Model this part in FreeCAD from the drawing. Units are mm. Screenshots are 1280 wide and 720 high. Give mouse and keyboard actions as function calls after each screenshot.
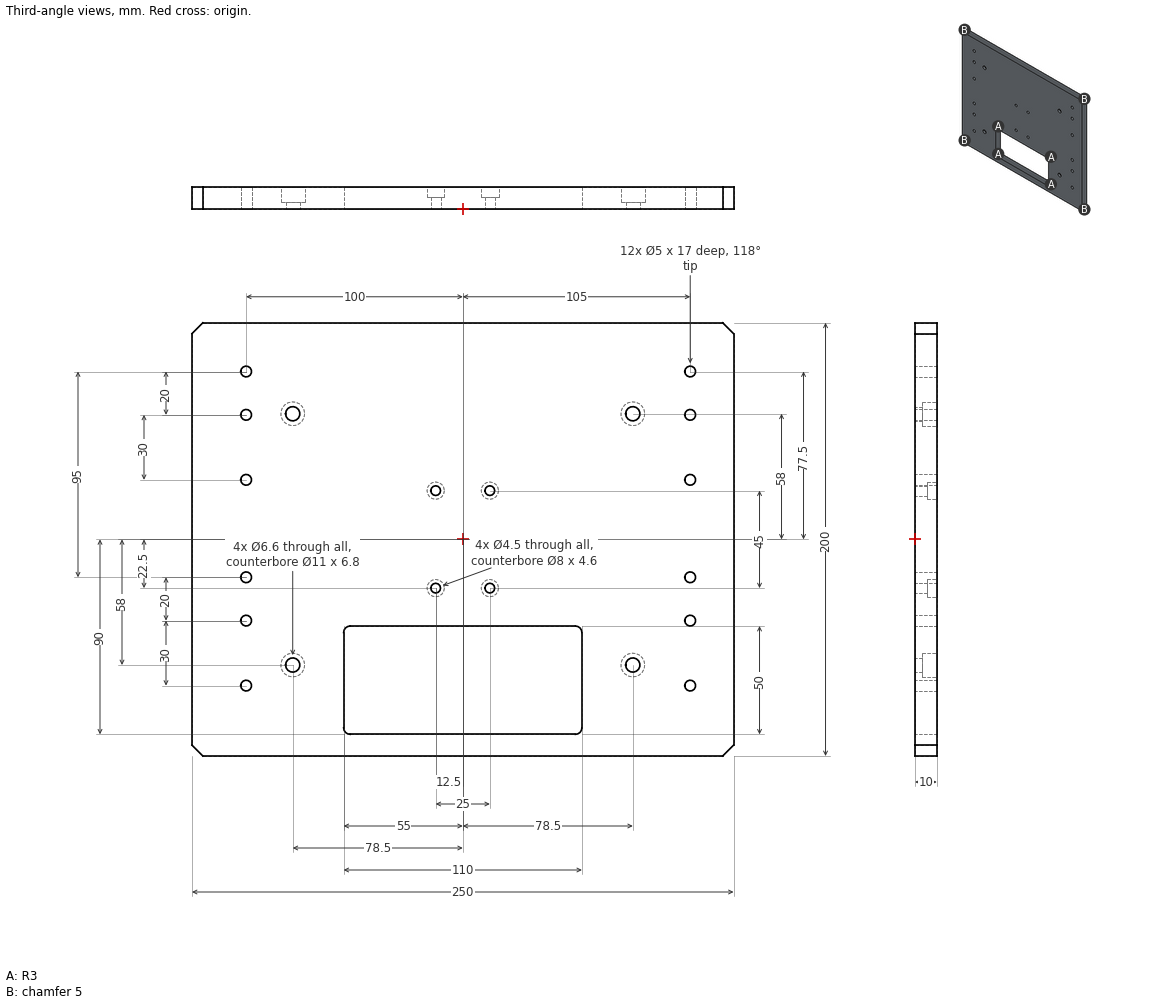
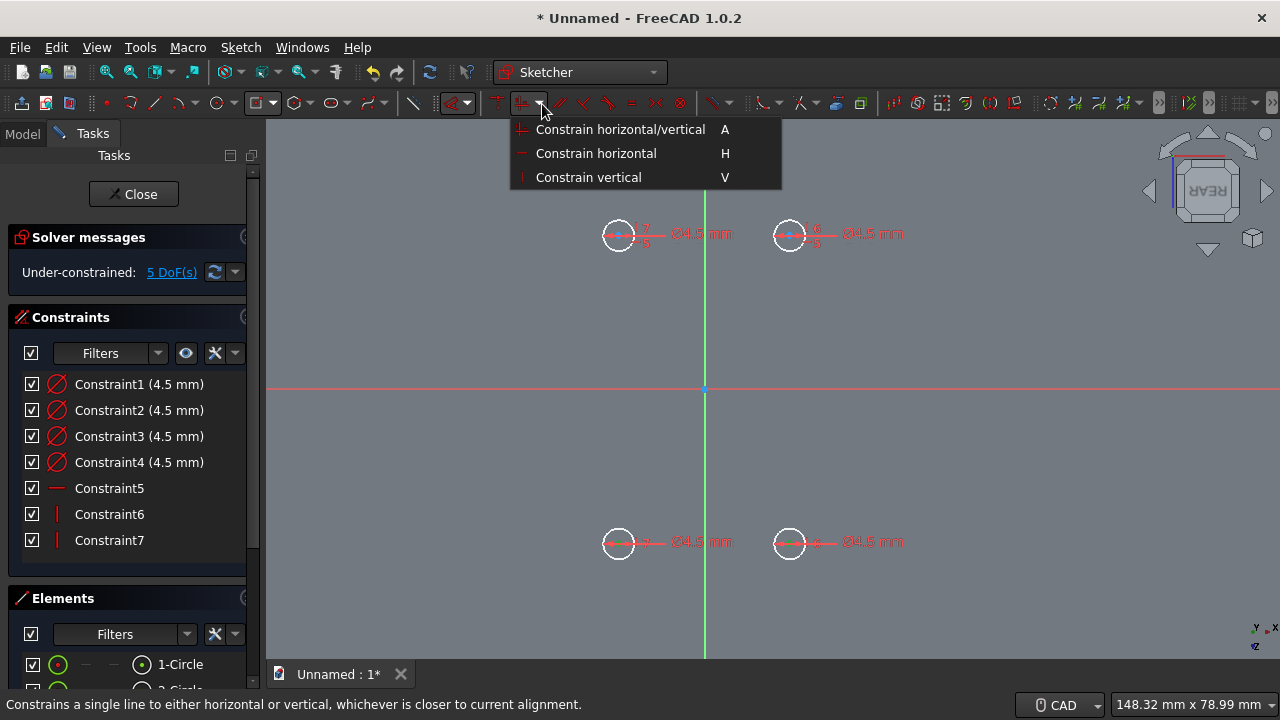
click(646, 153)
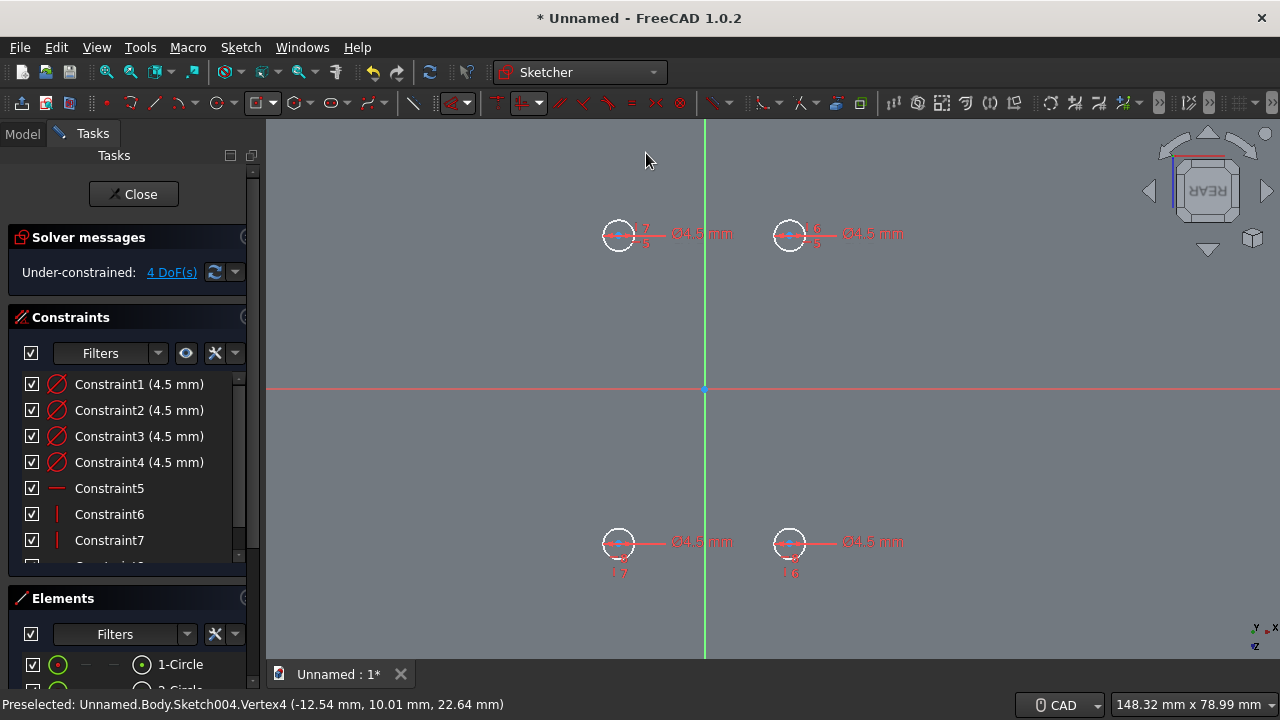
click(619, 236)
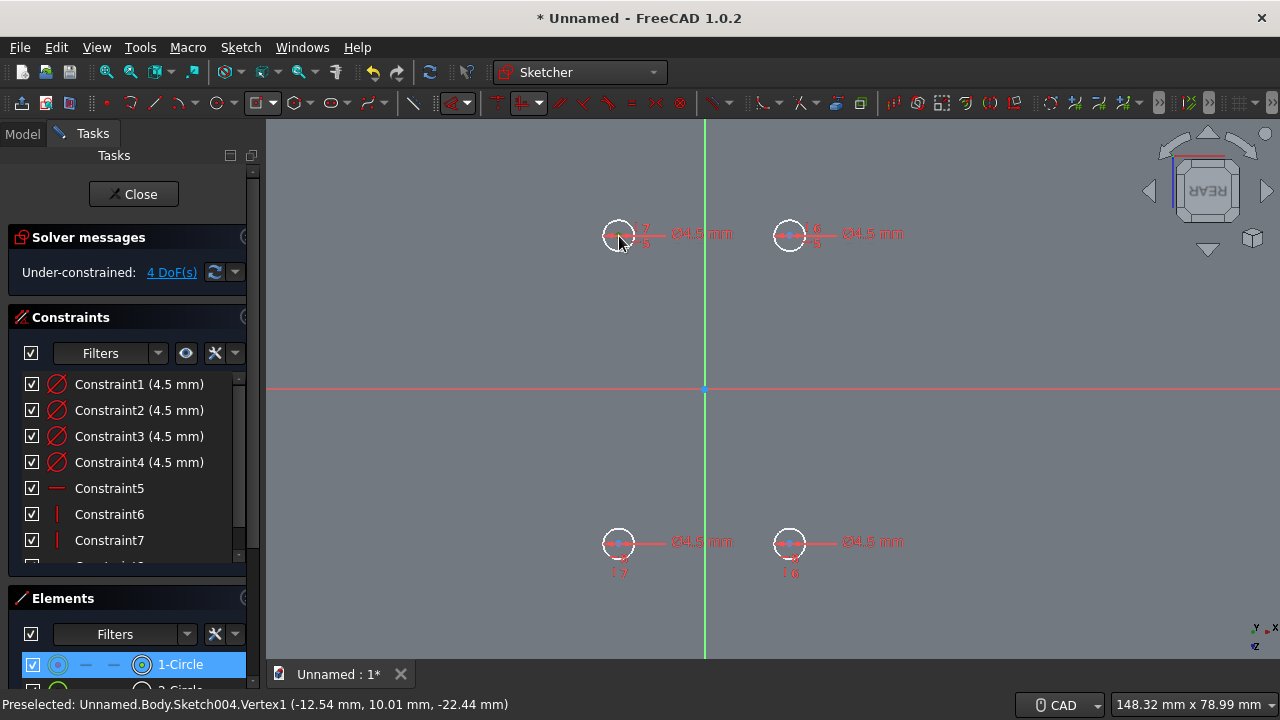
click(790, 236)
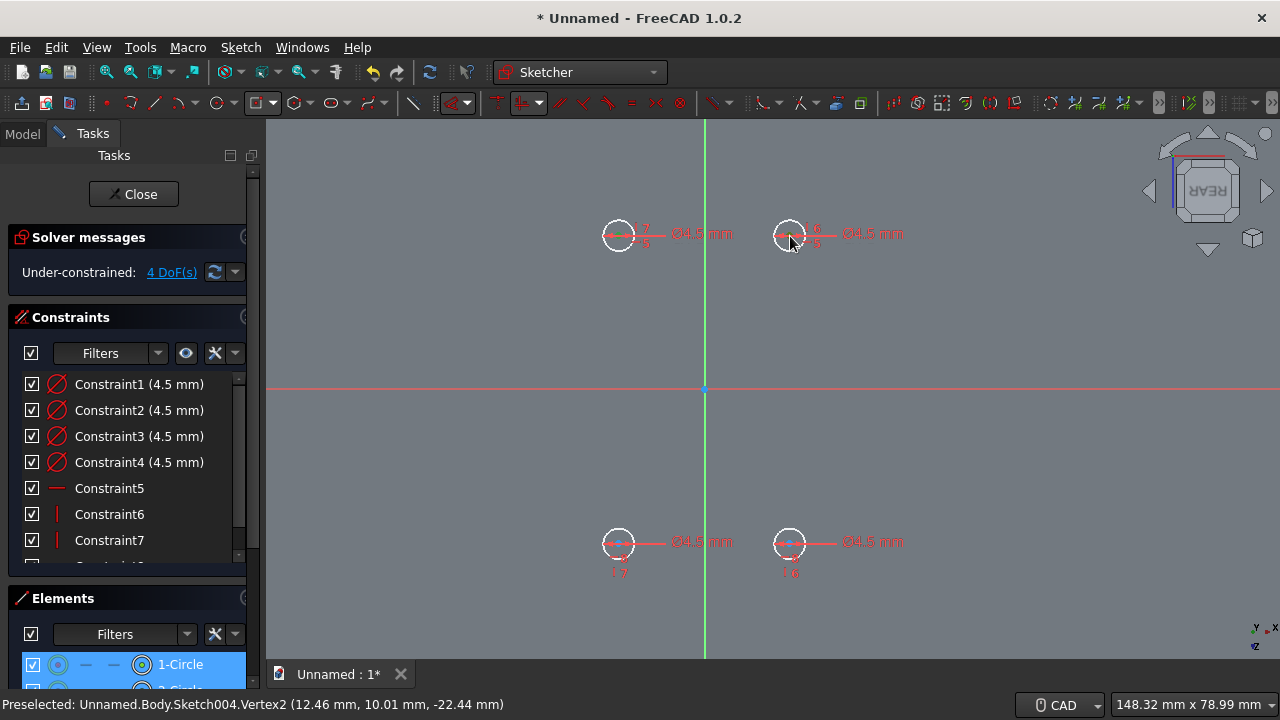
key(l)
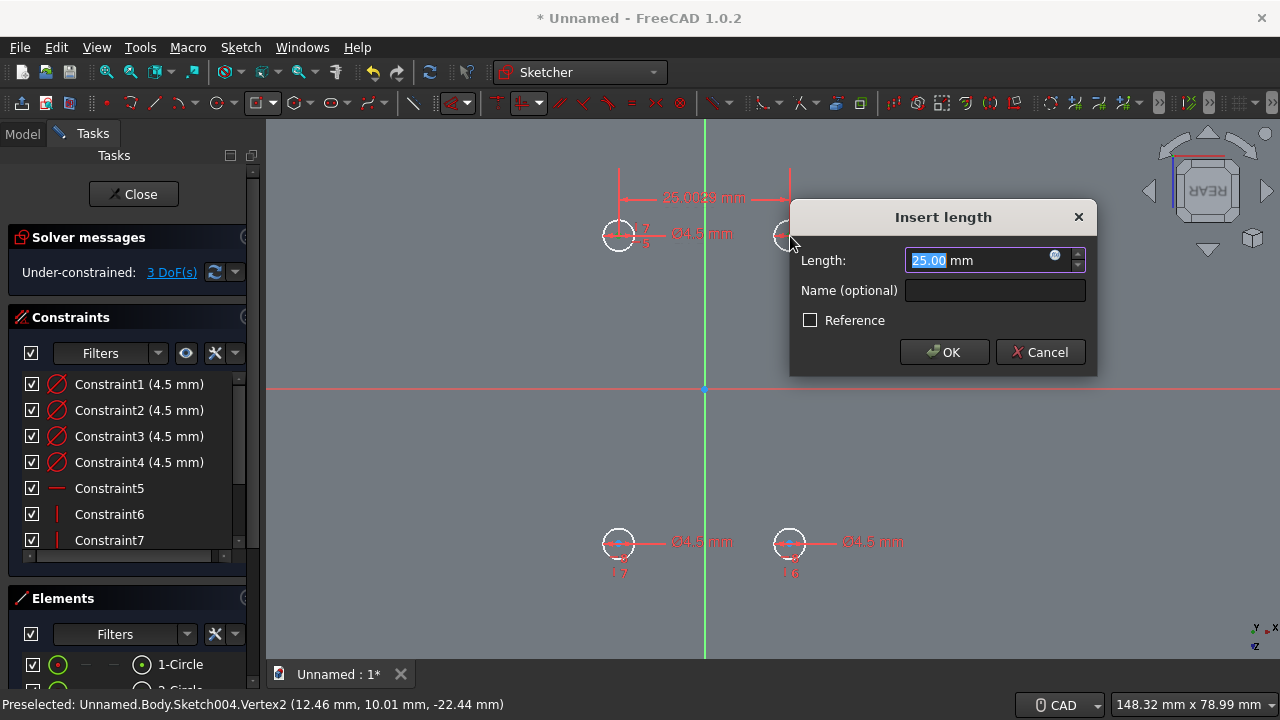
text(25)
key(Return)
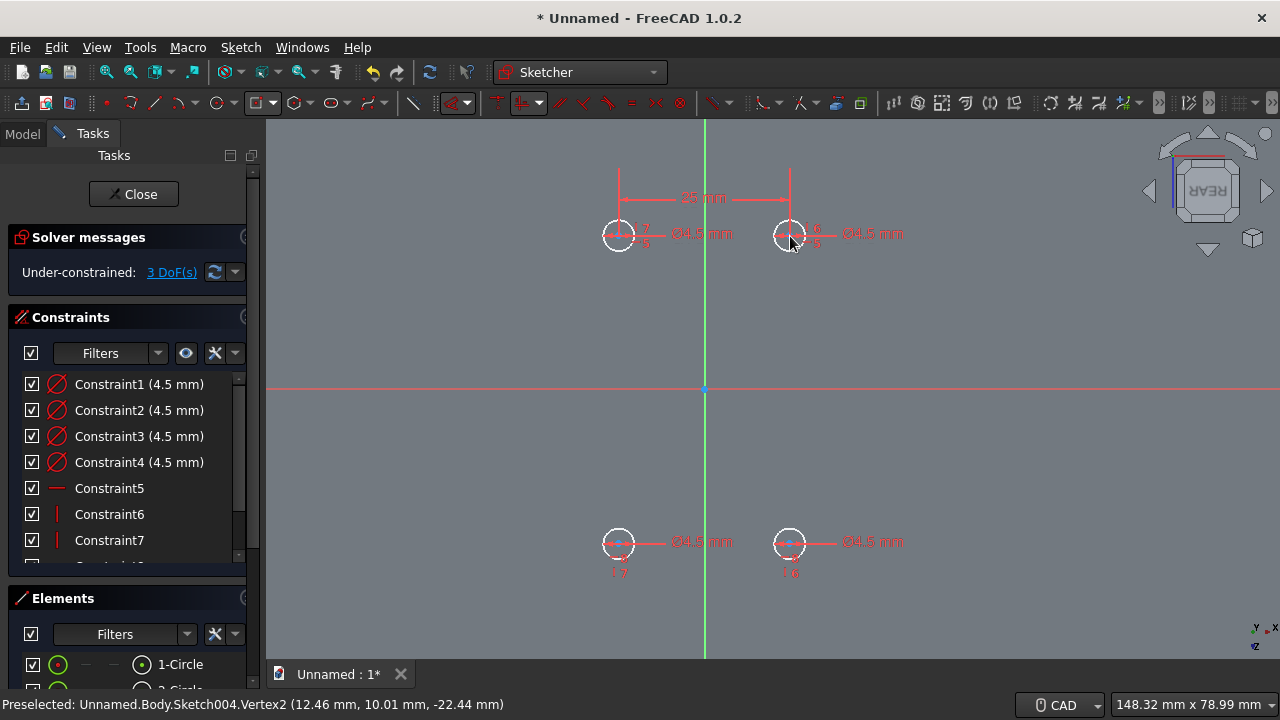
click(790, 236)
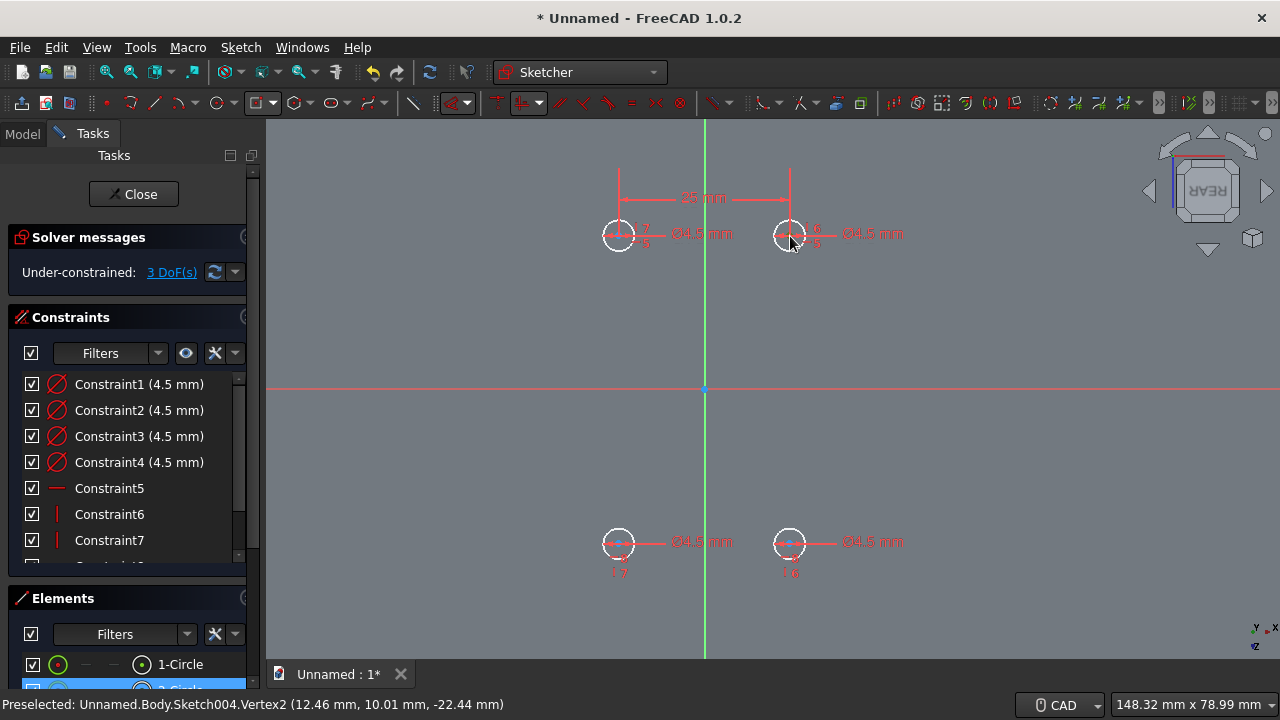
click(790, 544)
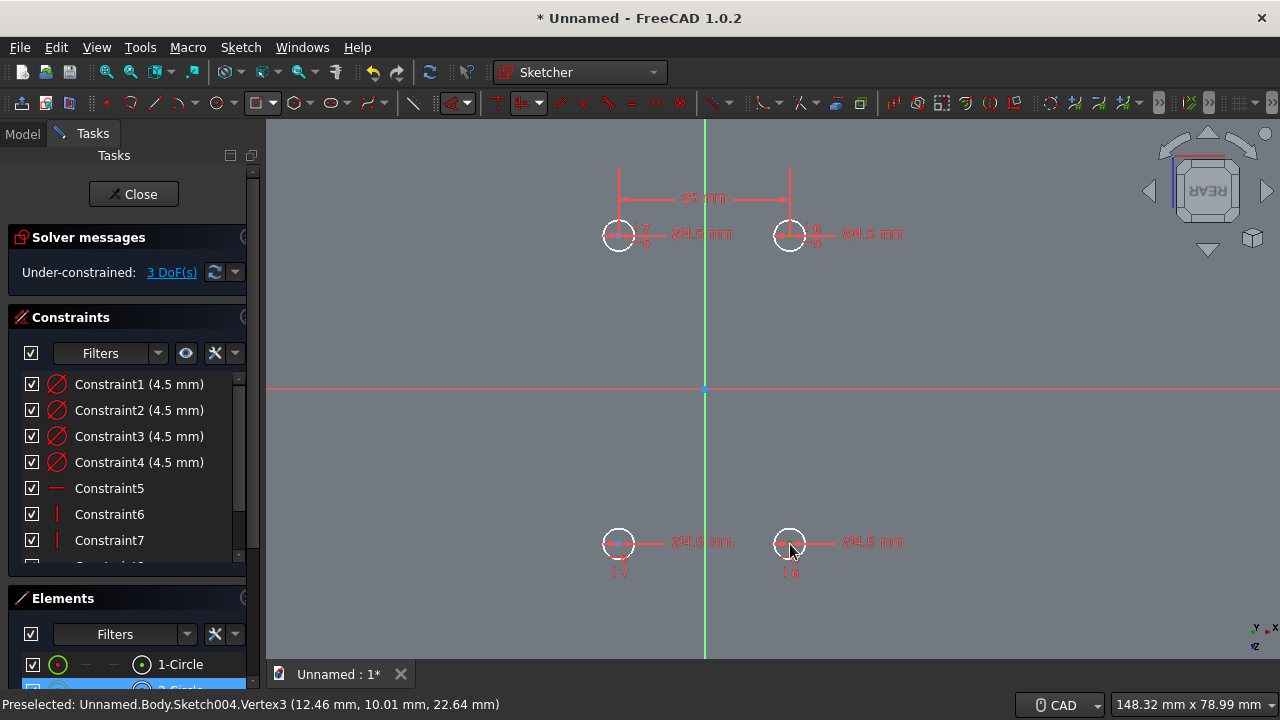
key(i)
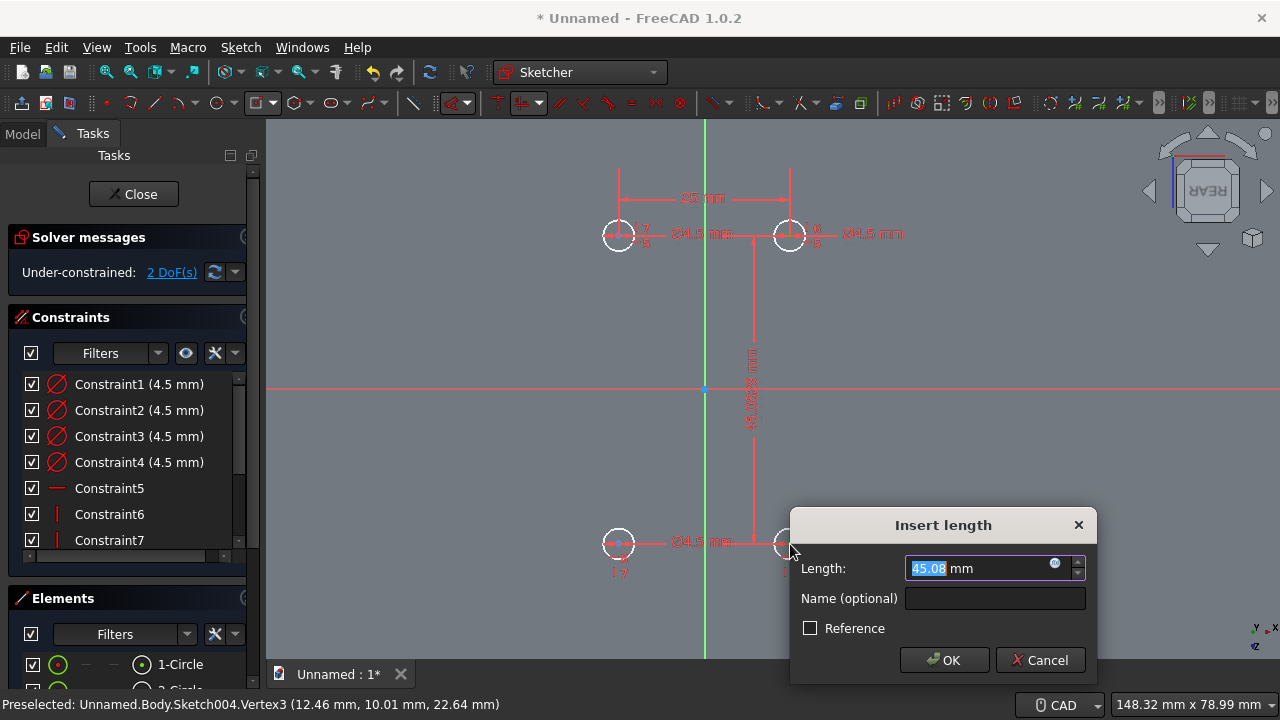
text(45)
key(Return)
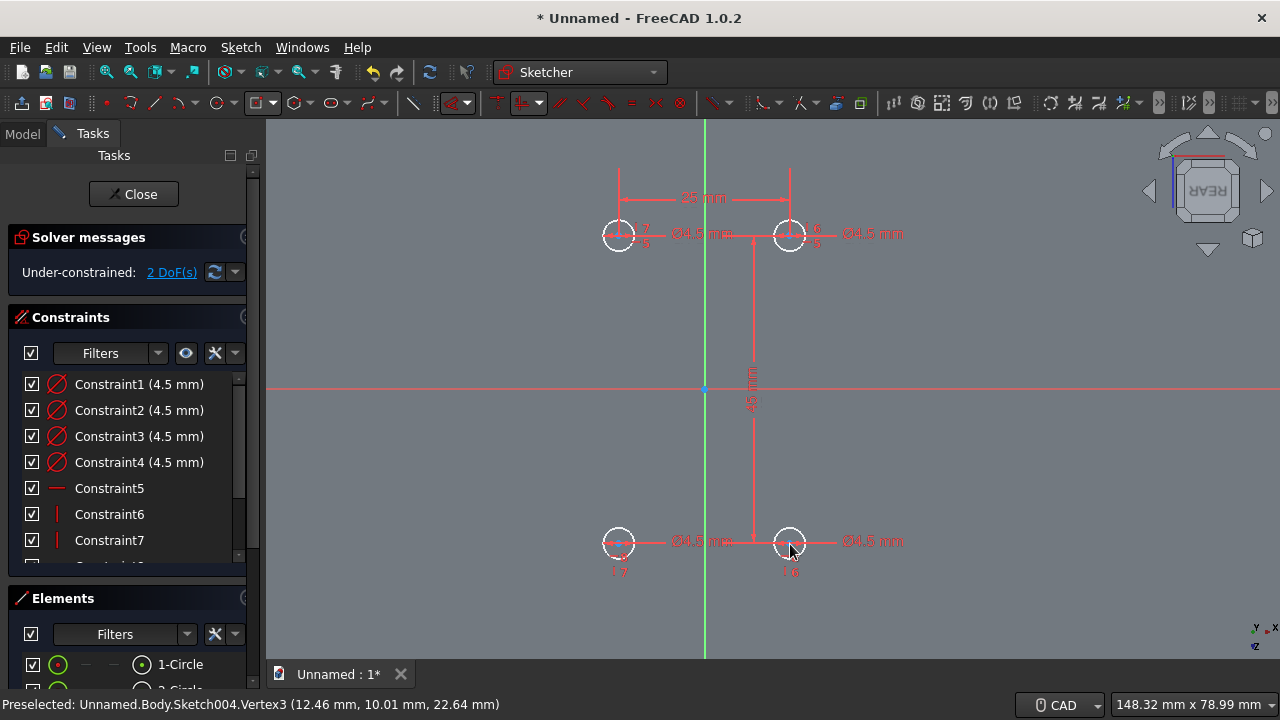
click(619, 236)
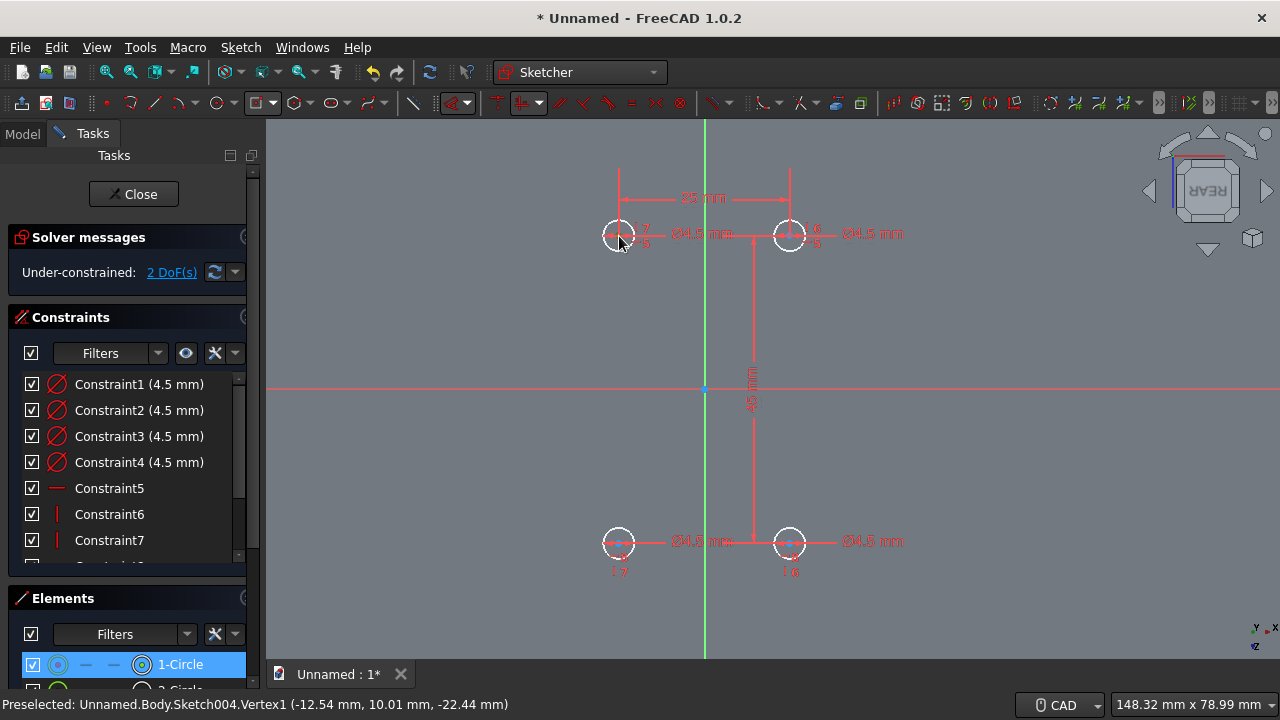
key(l)